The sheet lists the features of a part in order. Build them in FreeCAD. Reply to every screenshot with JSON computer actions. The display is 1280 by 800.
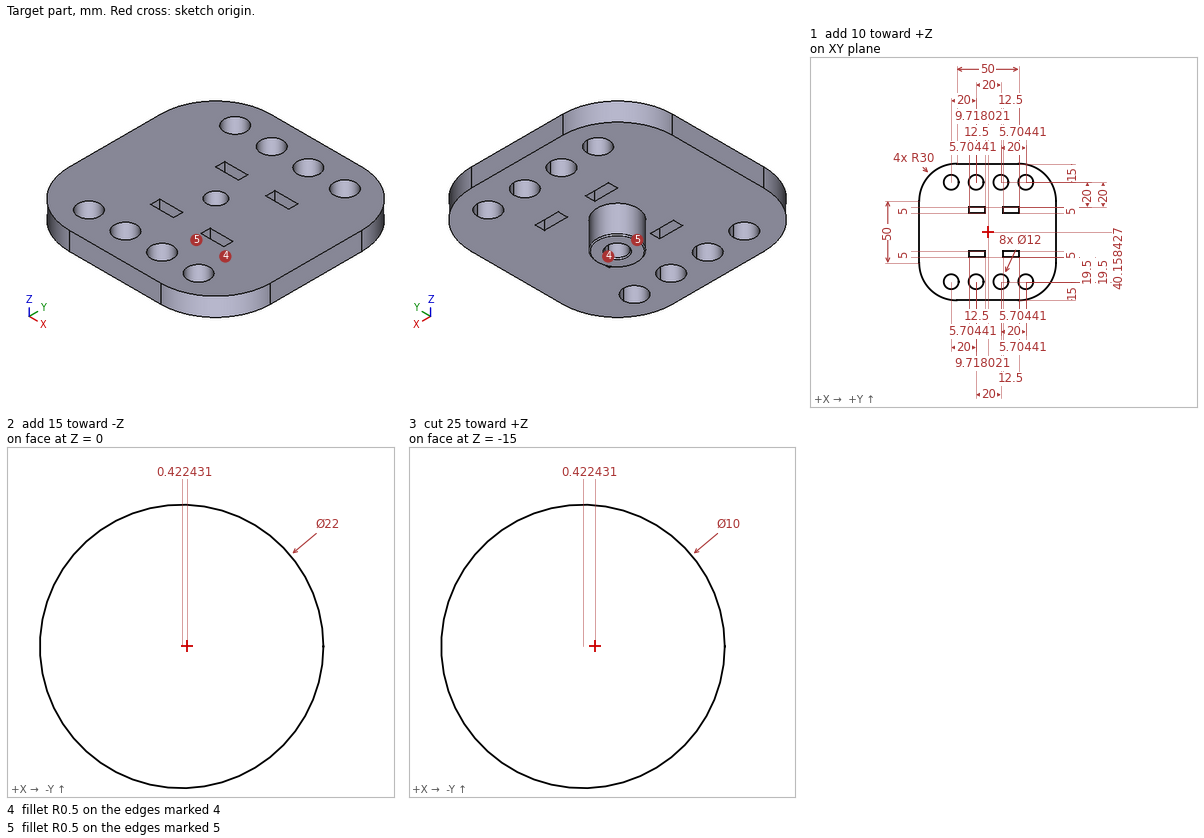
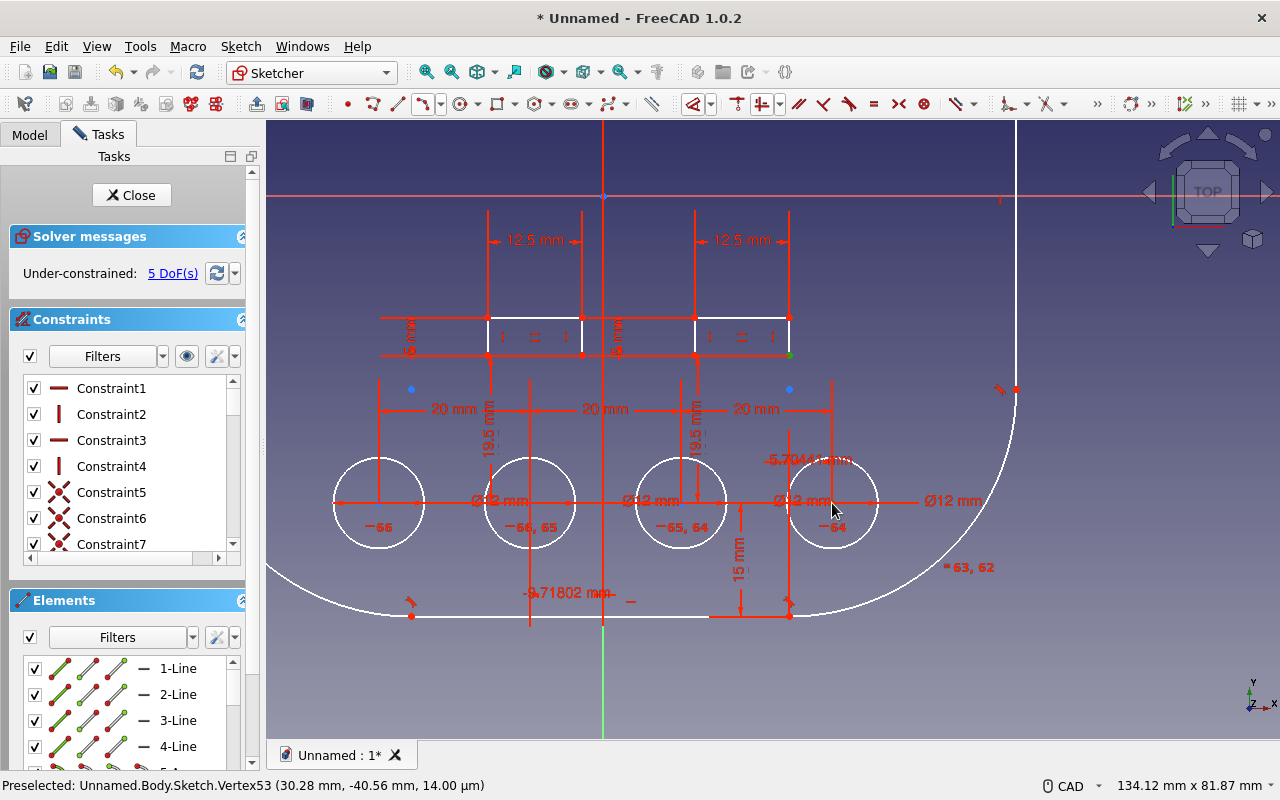
{"action": "left_click", "coordinate": [710, 104]}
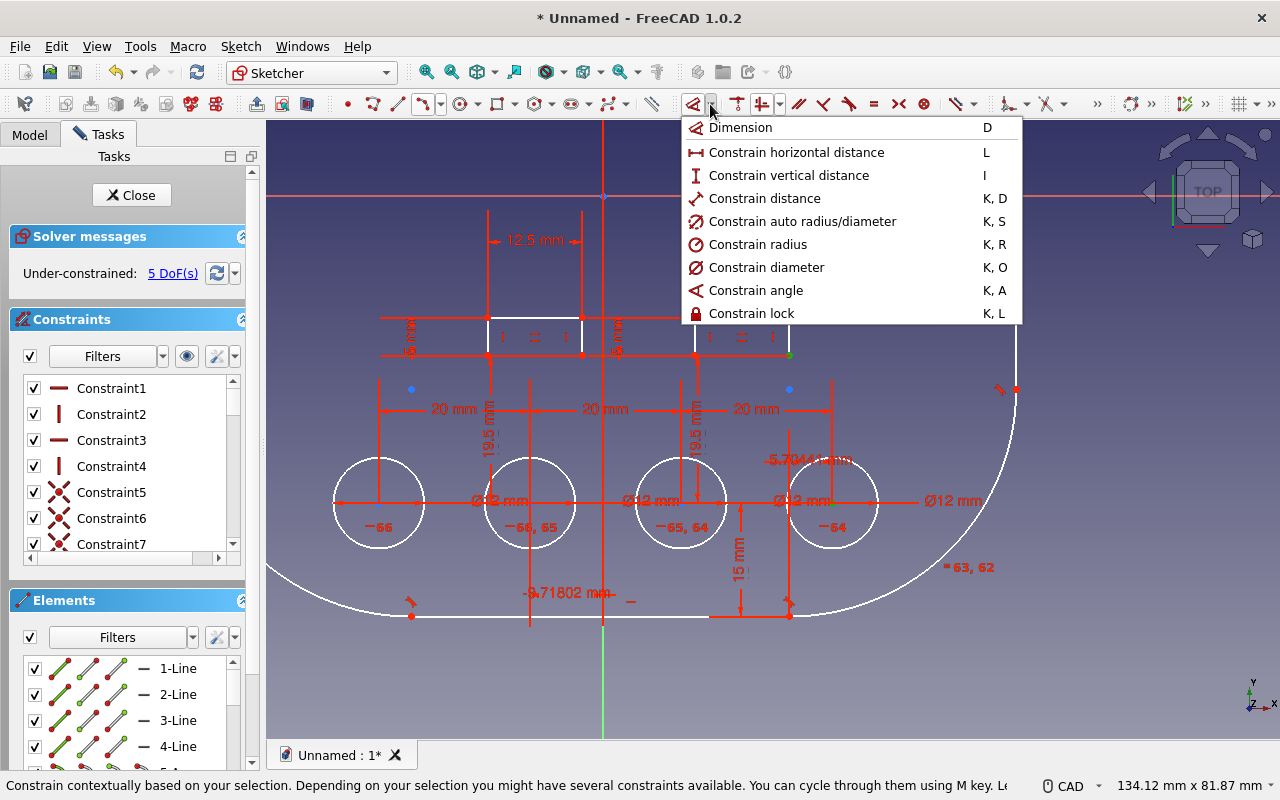
{"action": "left_click", "coordinate": [852, 152]}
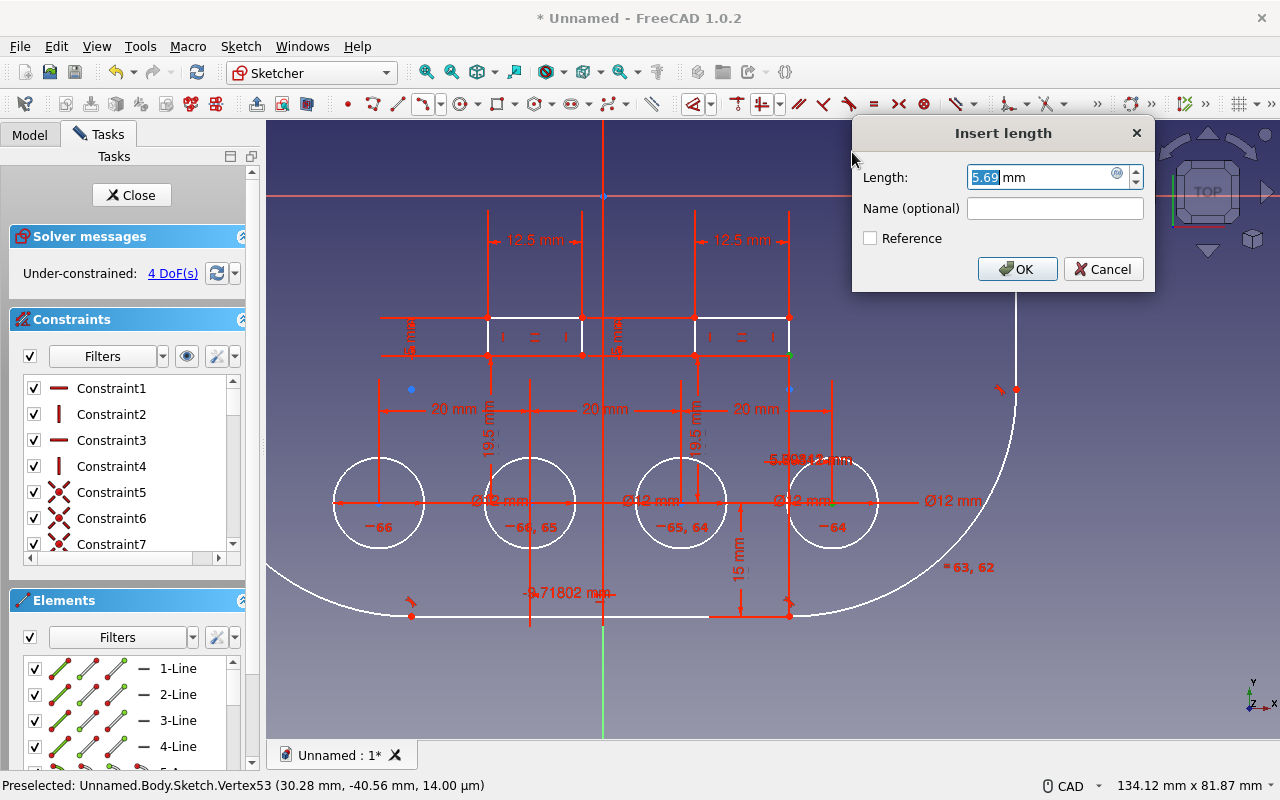
{"action": "type", "text": "5.70441"}
{"action": "key", "text": "Return"}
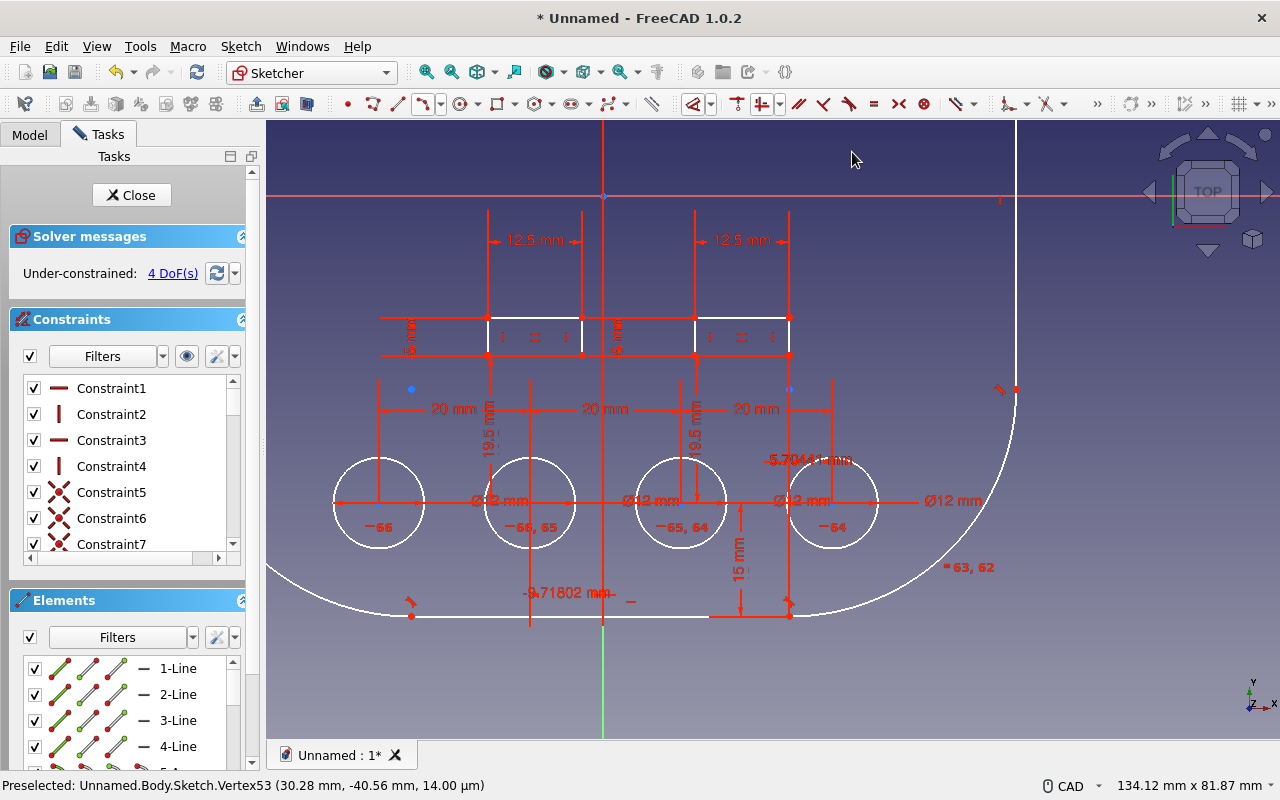
{"action": "left_click", "coordinate": [488, 356]}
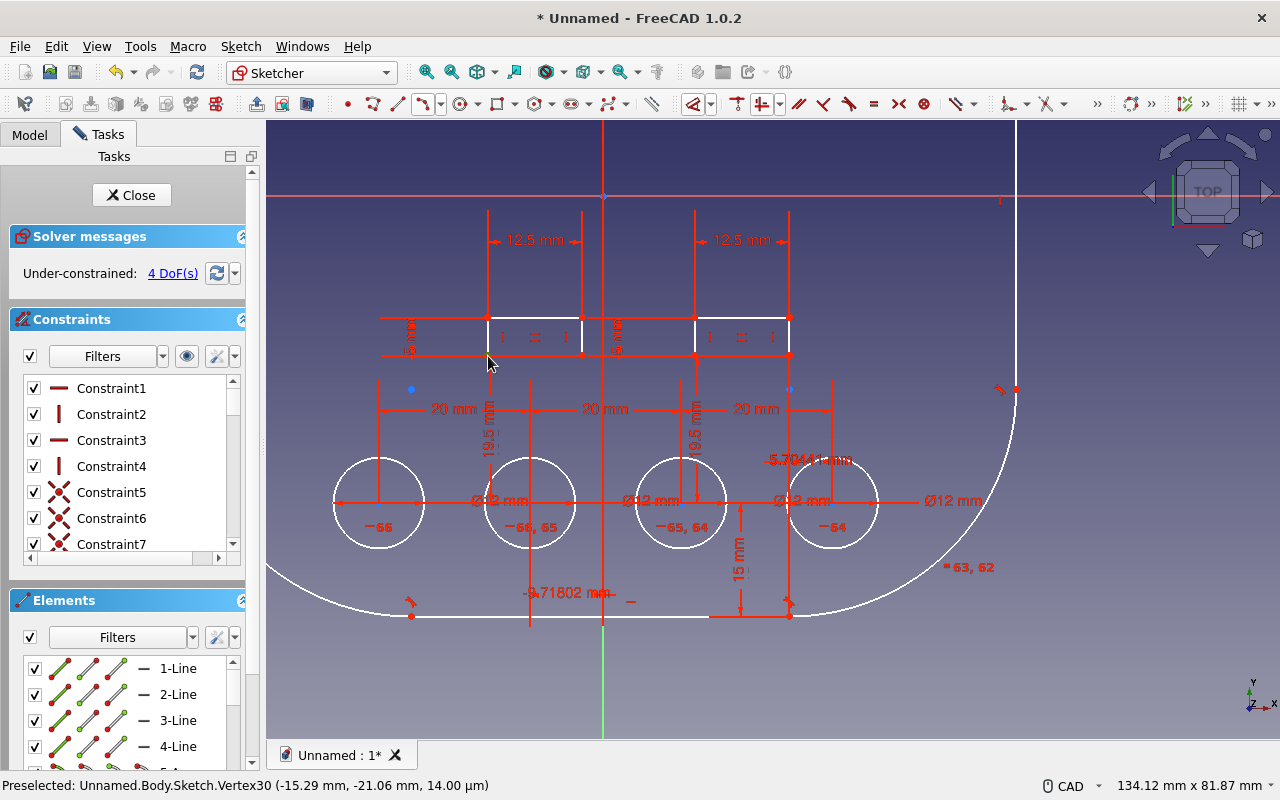
{"action": "left_click", "coordinate": [530, 503]}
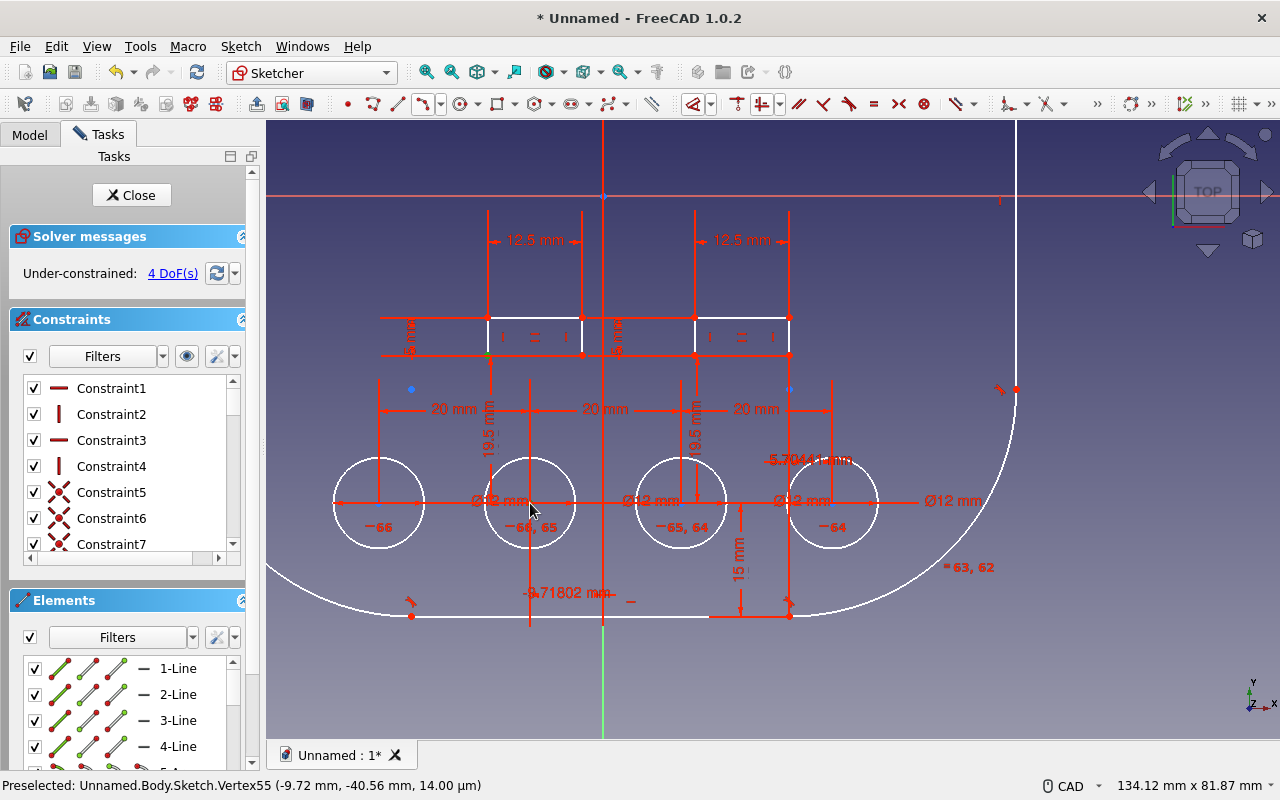
{"action": "left_click", "coordinate": [710, 104]}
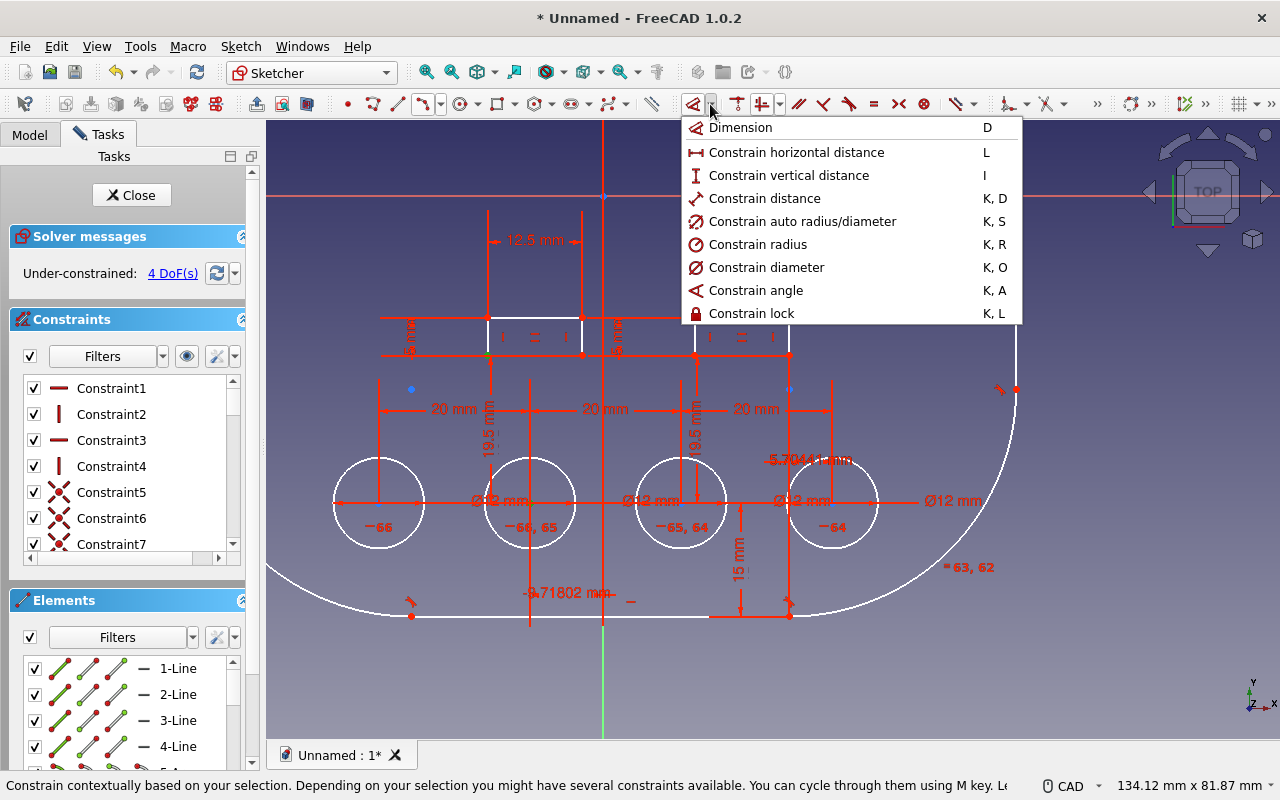
{"action": "left_click", "coordinate": [852, 152]}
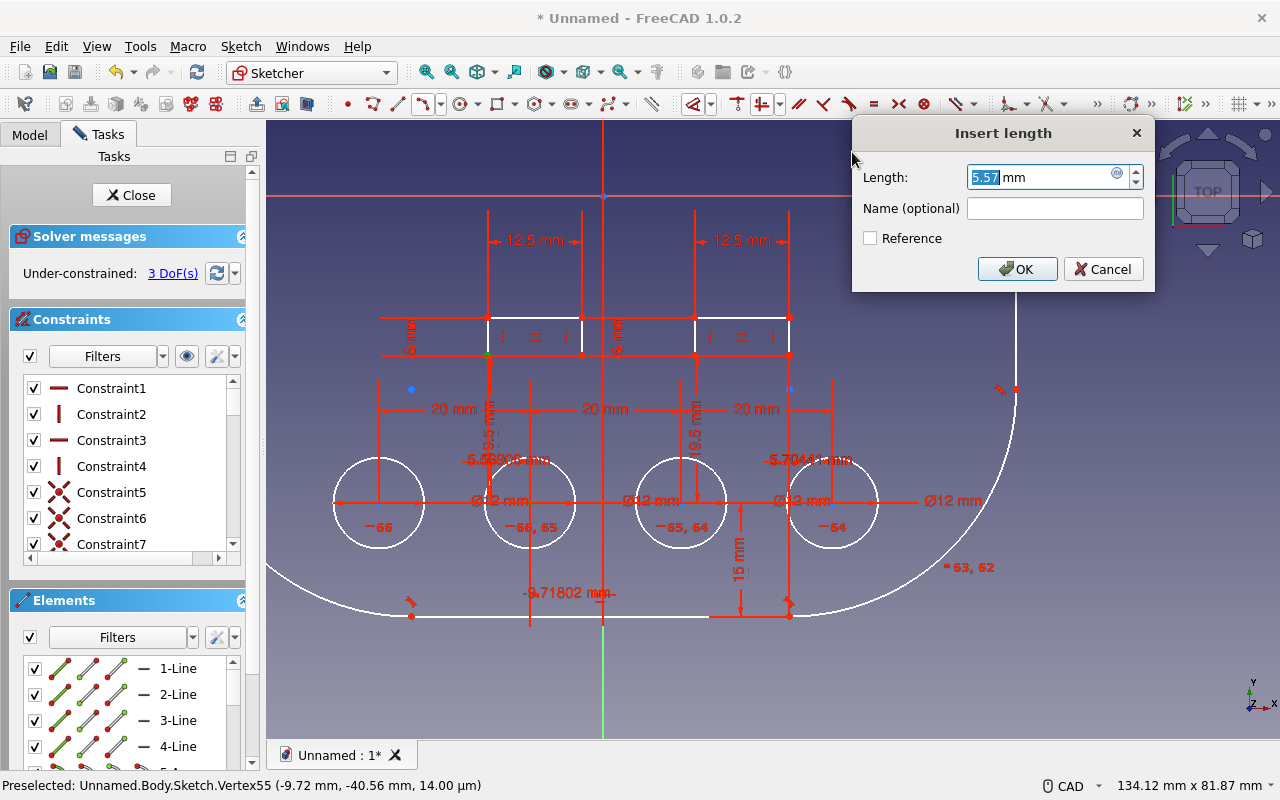
{"action": "type", "text": "5.70441"}
{"action": "key", "text": "Return"}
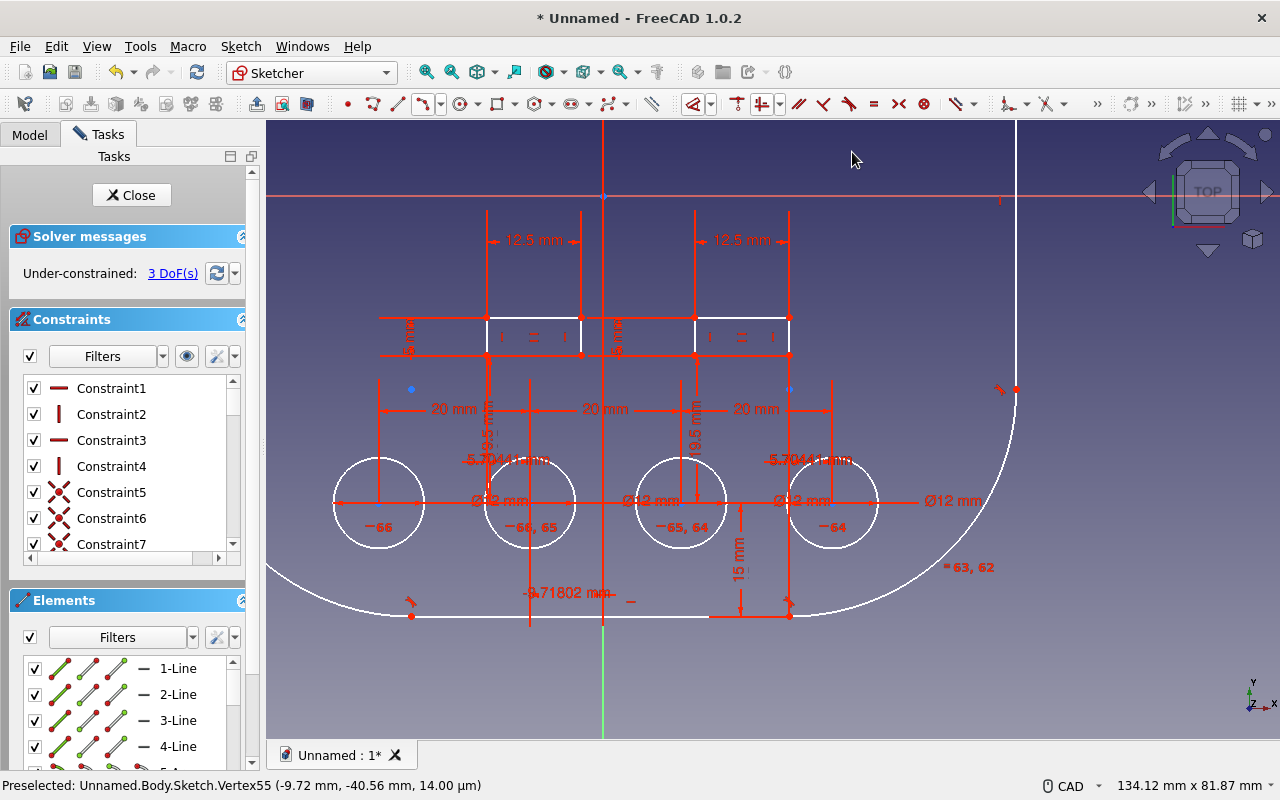
{"action": "scroll", "coordinate": [790, 619], "scroll_direction": "down", "scroll_amount": 4}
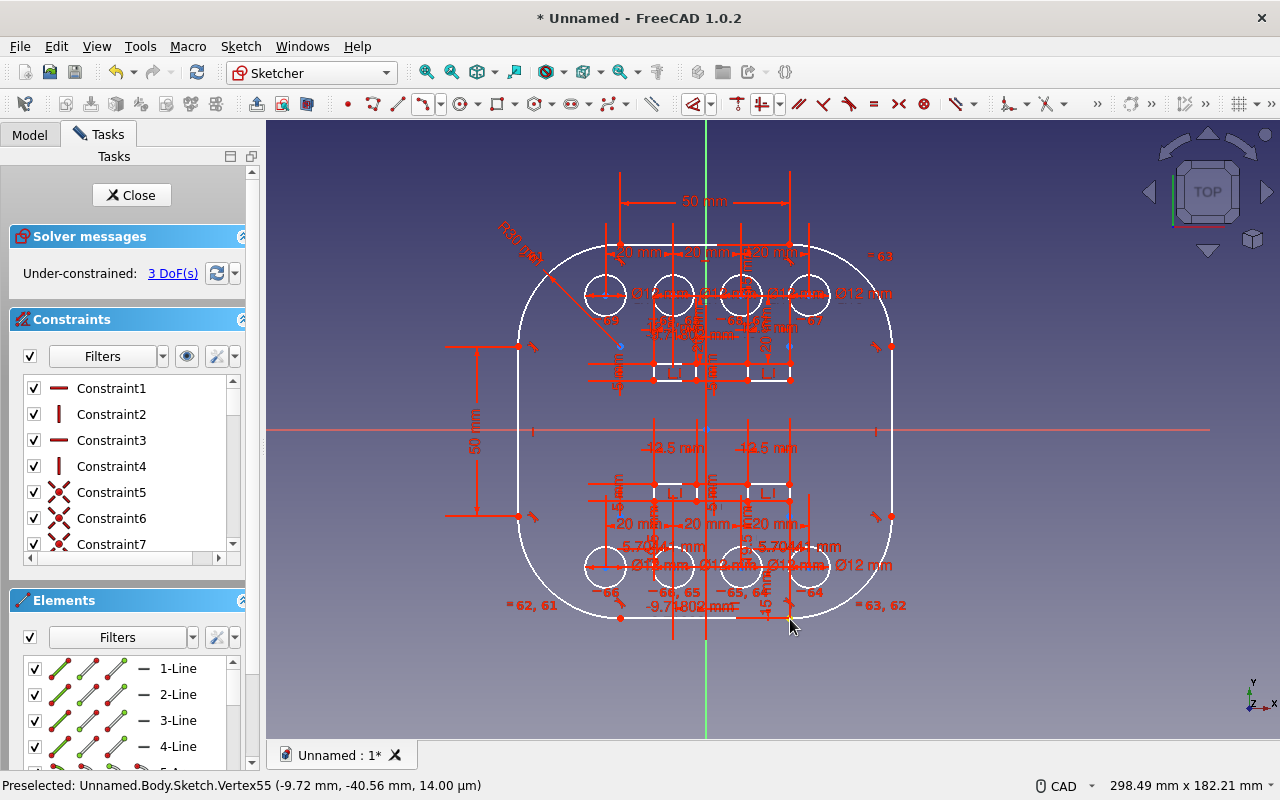
{"action": "scroll", "coordinate": [790, 364], "scroll_direction": "up", "scroll_amount": 4}